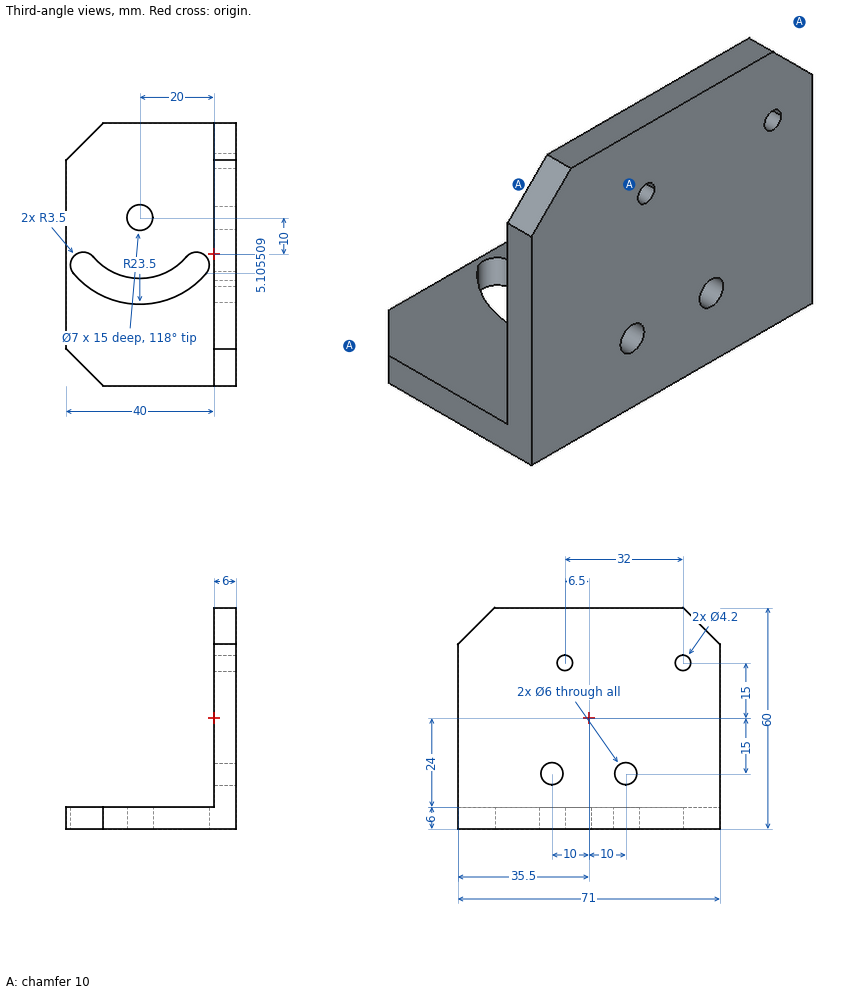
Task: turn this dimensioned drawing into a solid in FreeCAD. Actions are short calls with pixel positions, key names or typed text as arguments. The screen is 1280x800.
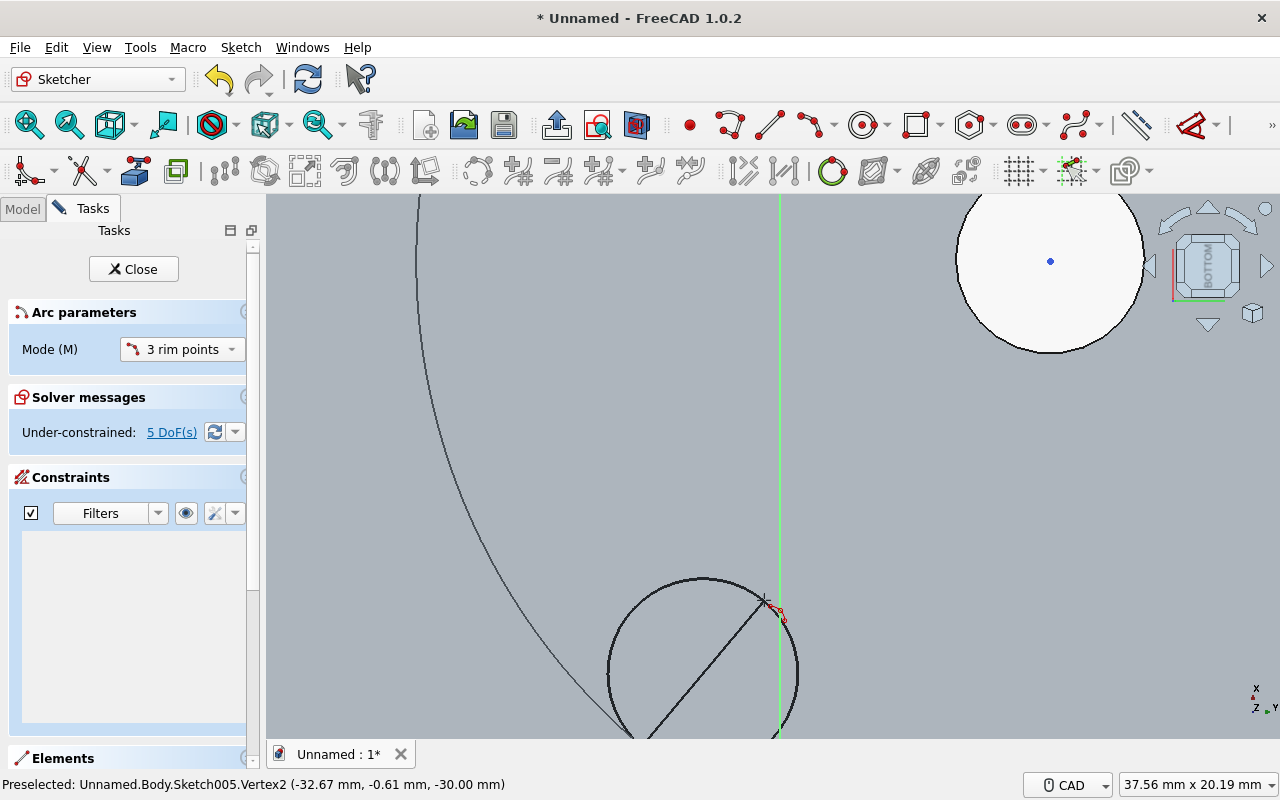
scroll(766, 603, down, 5)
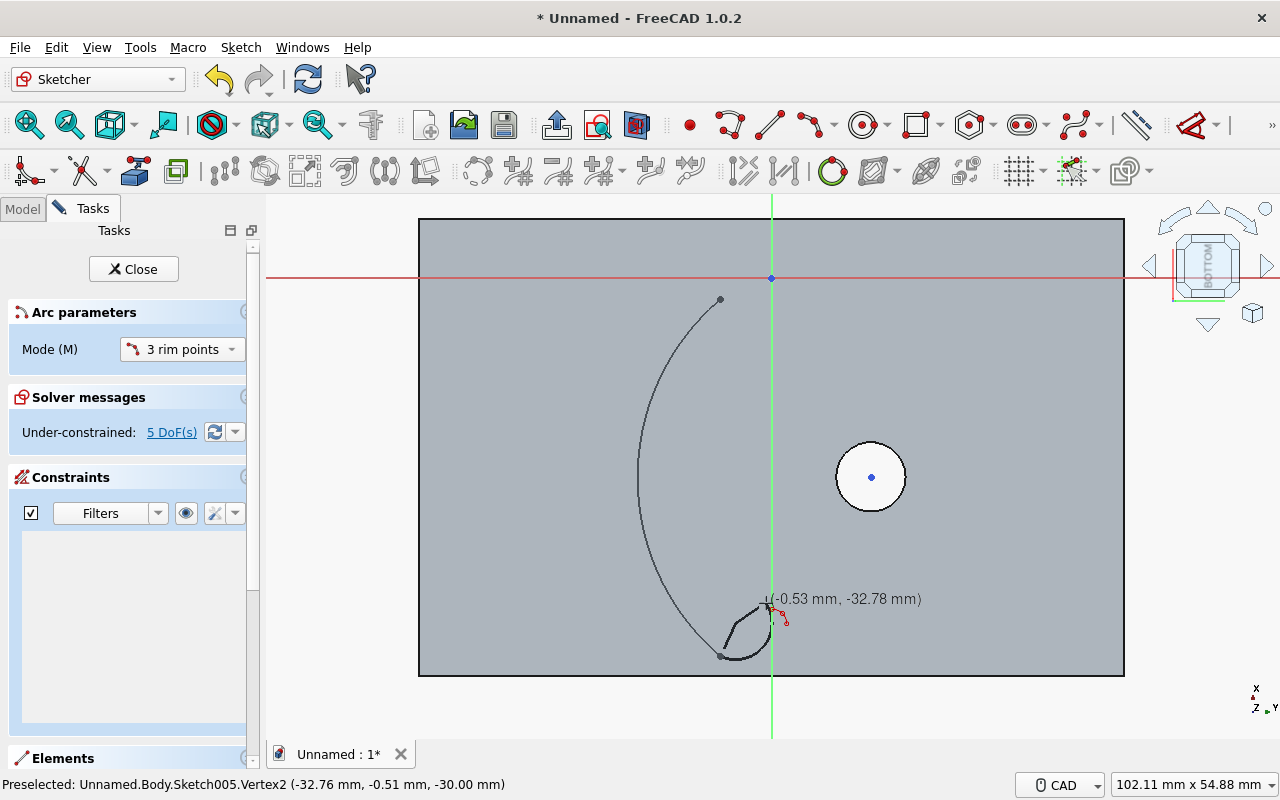
click(752, 663)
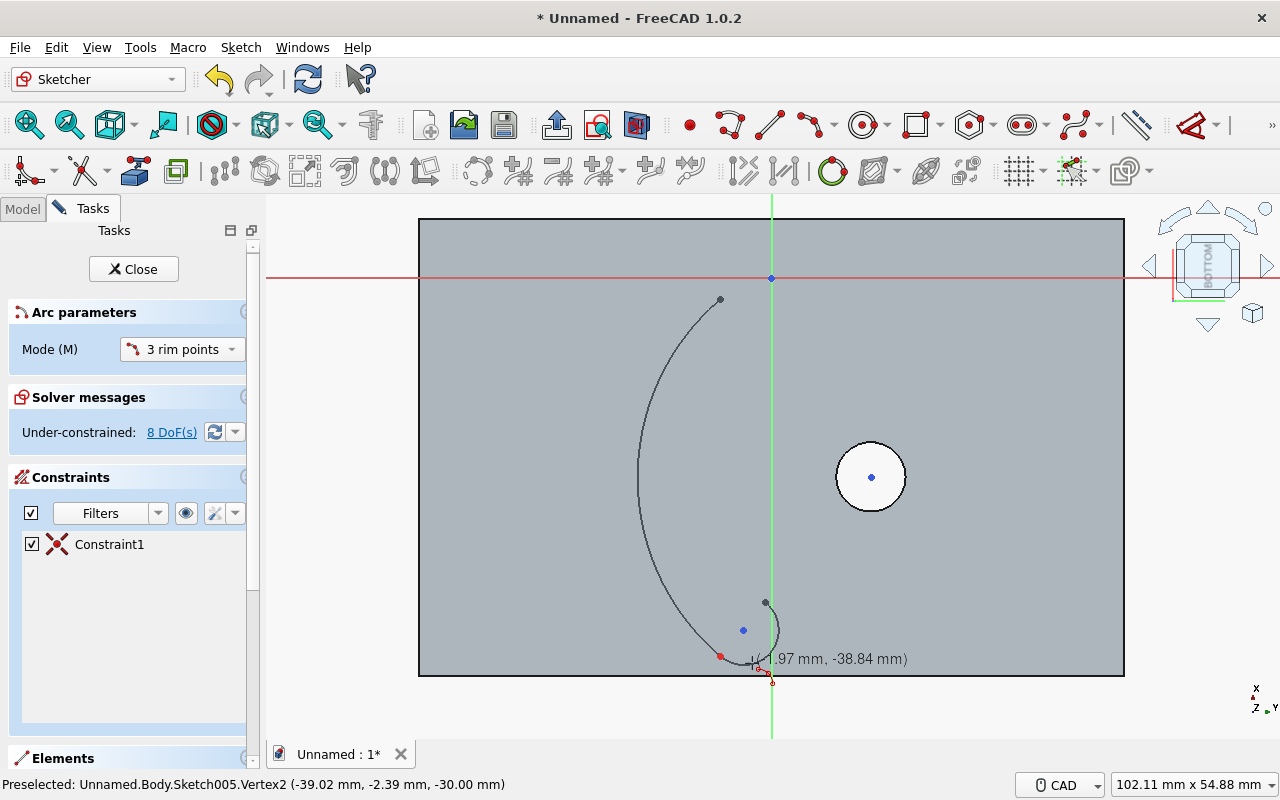
scroll(766, 602, up, 5)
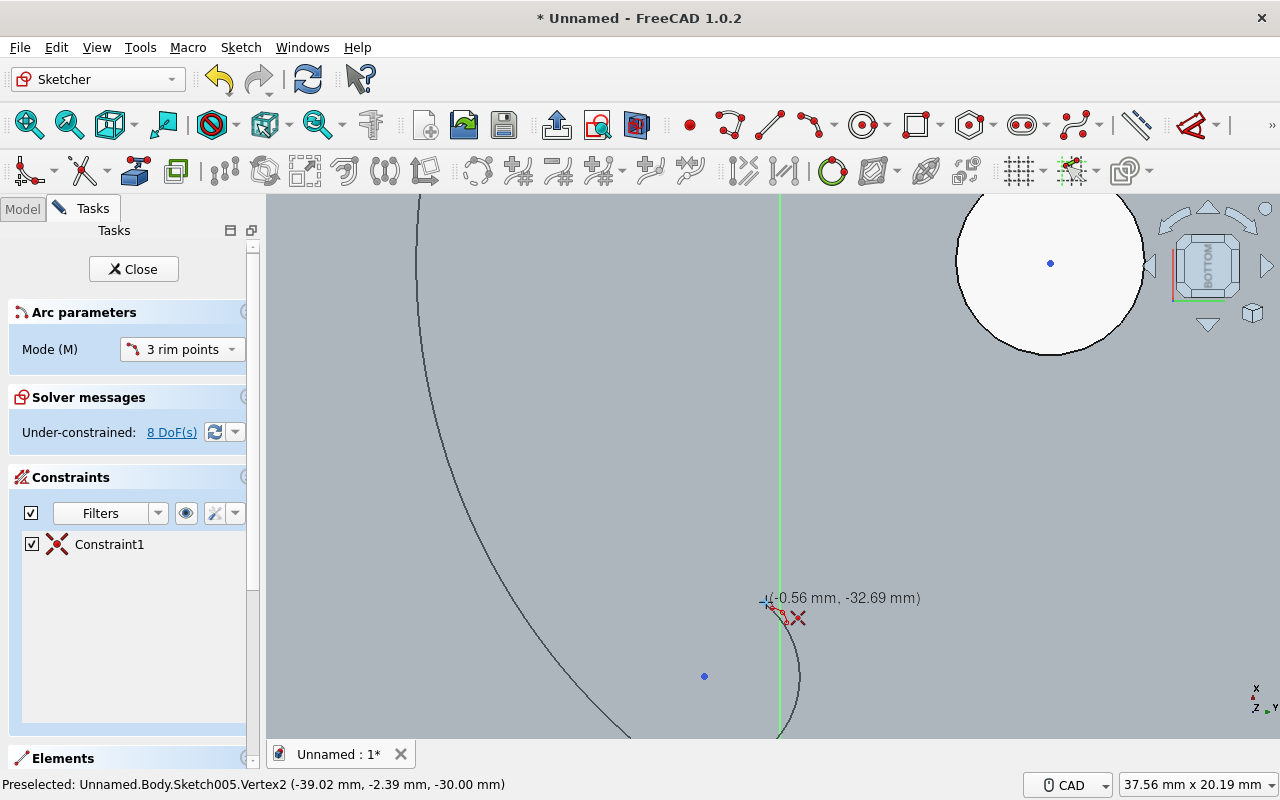
click(764, 603)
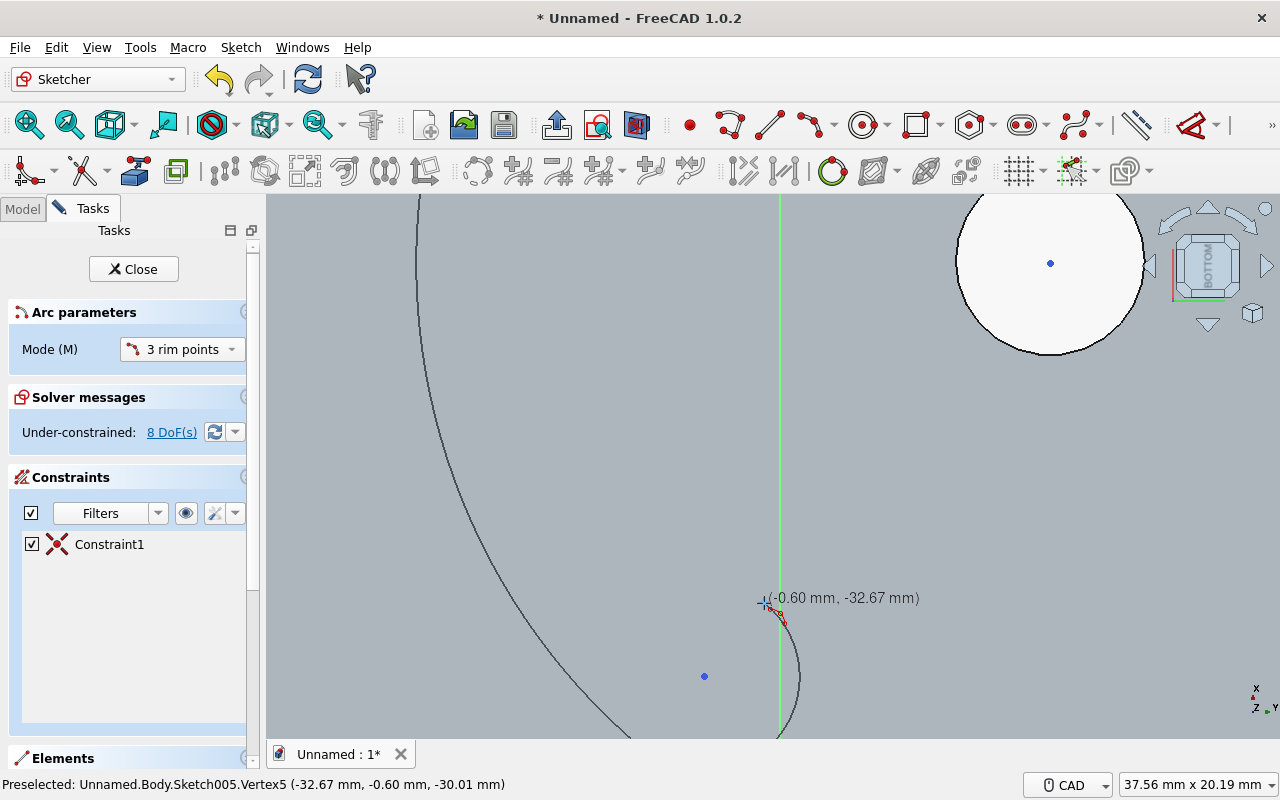
scroll(766, 602, down, 5)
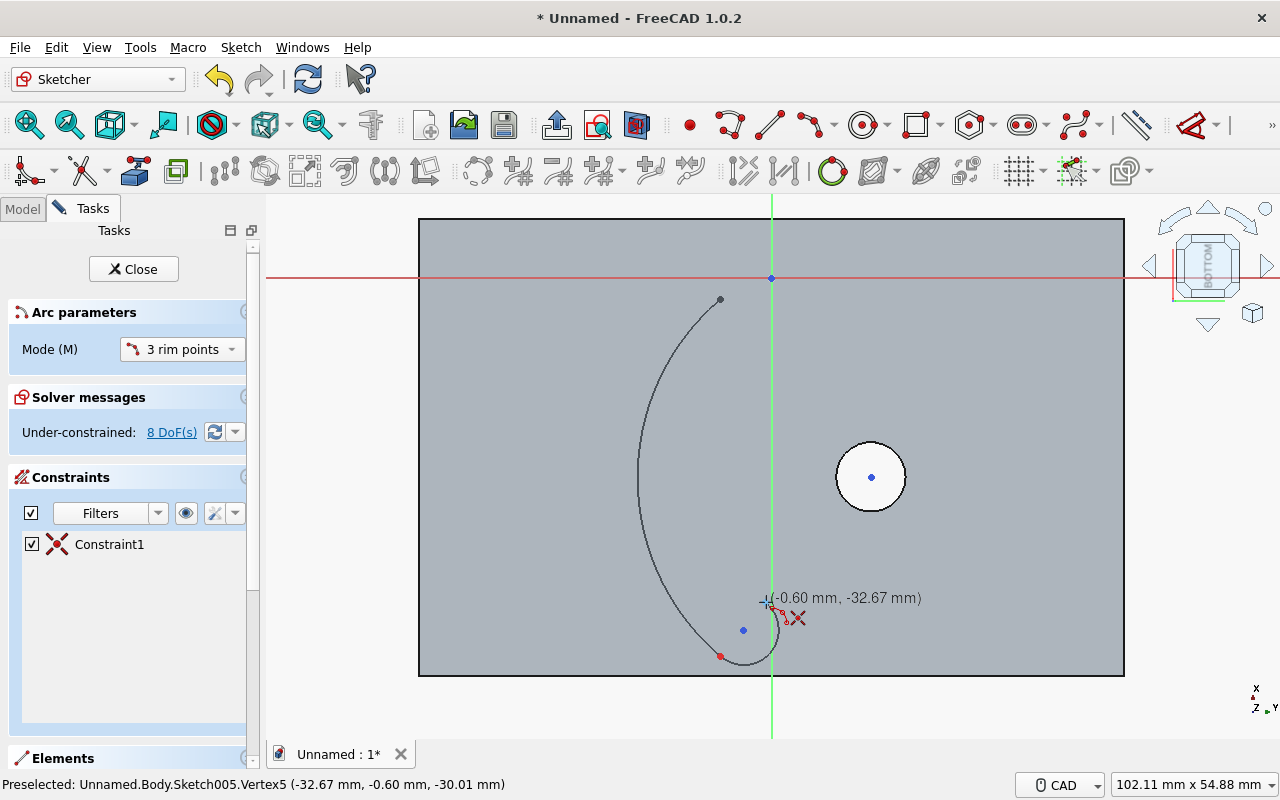
scroll(766, 351, up, 5)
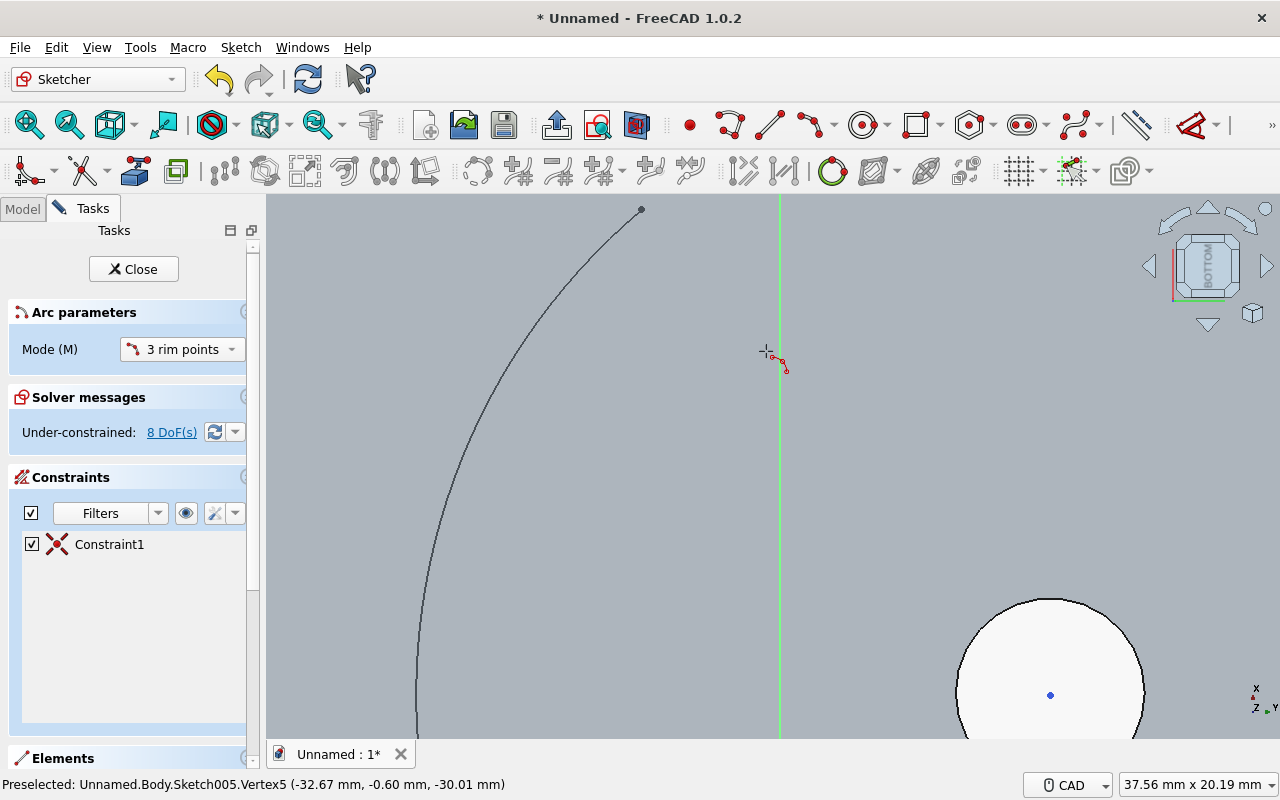
click(764, 352)
click(605, 693)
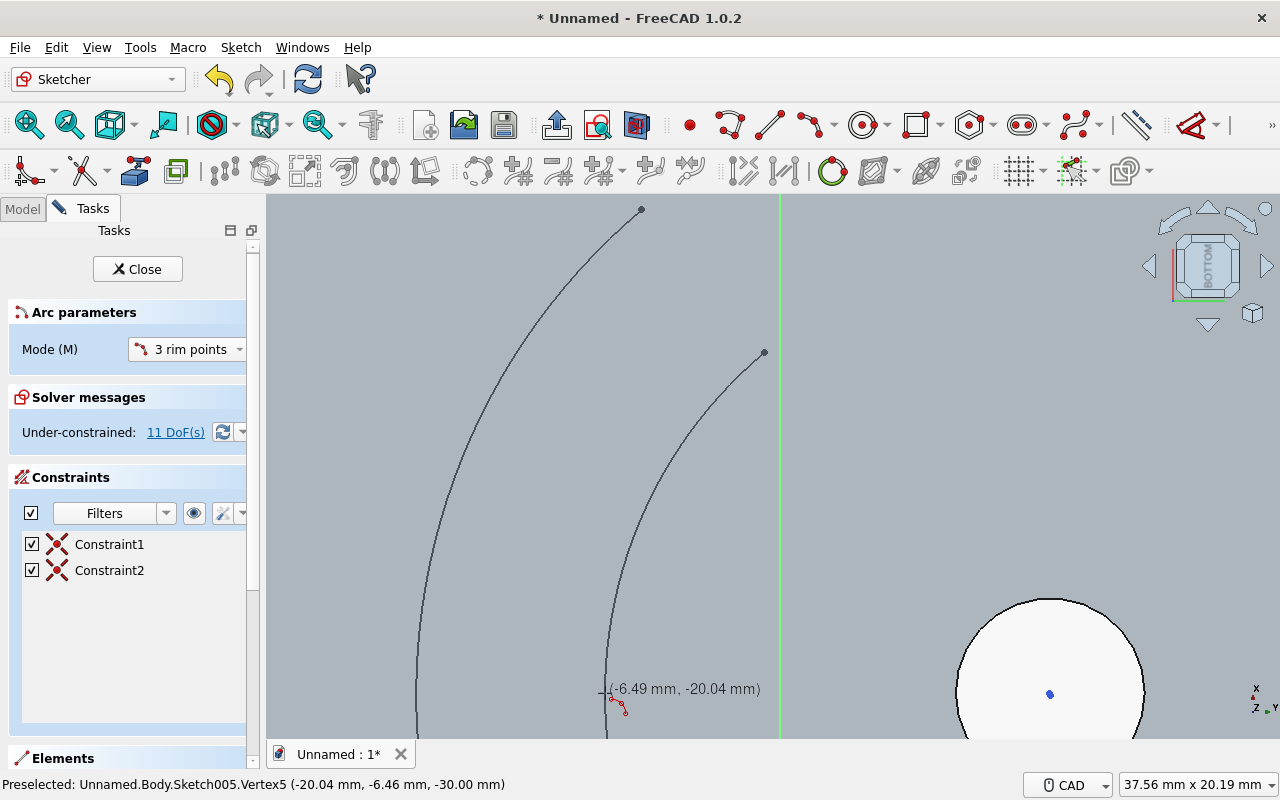
click(764, 353)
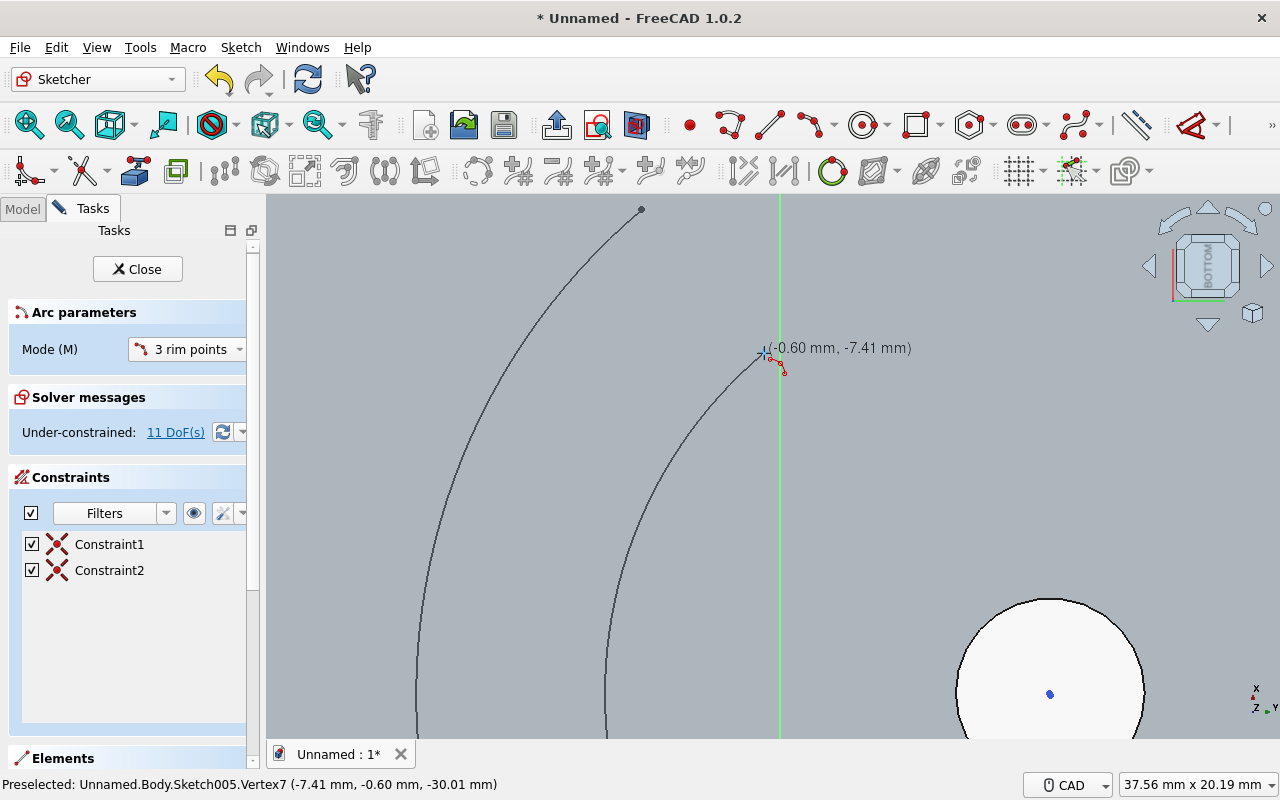
scroll(766, 350, down, 5)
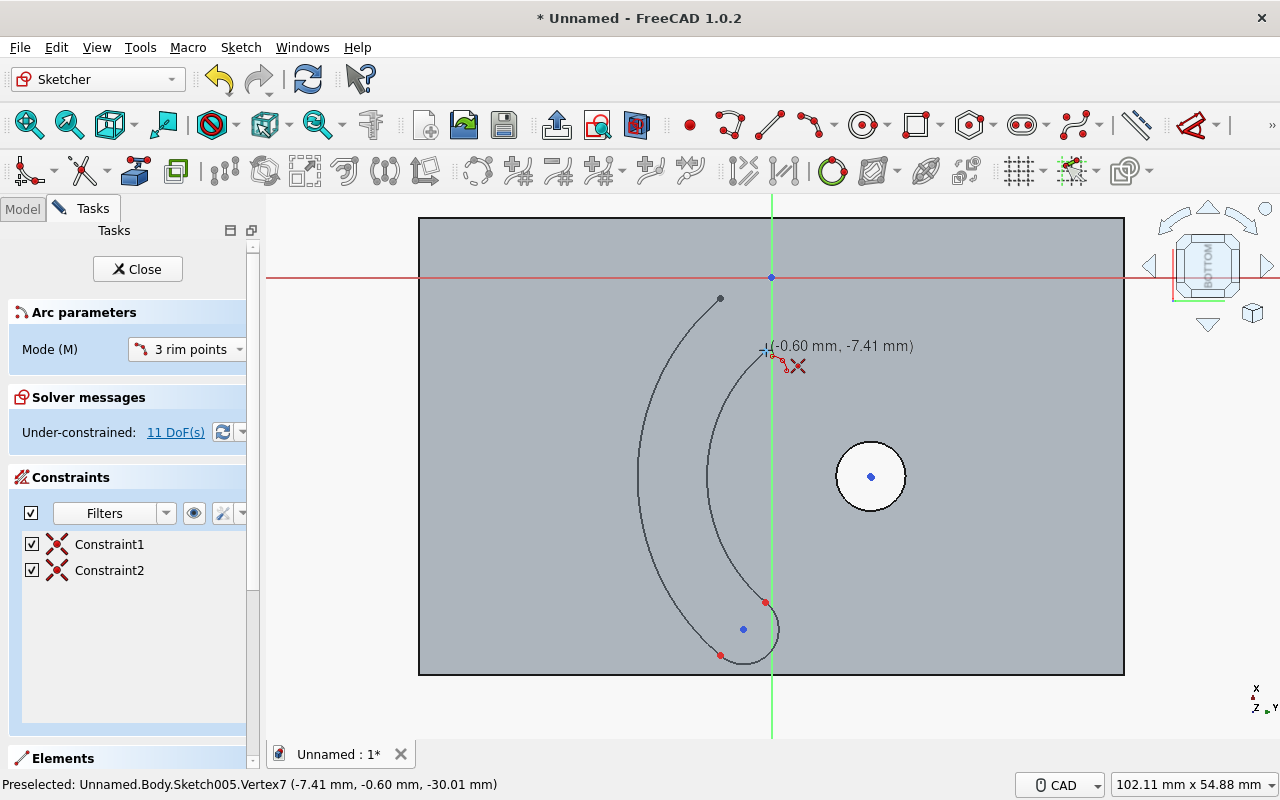
click(721, 299)